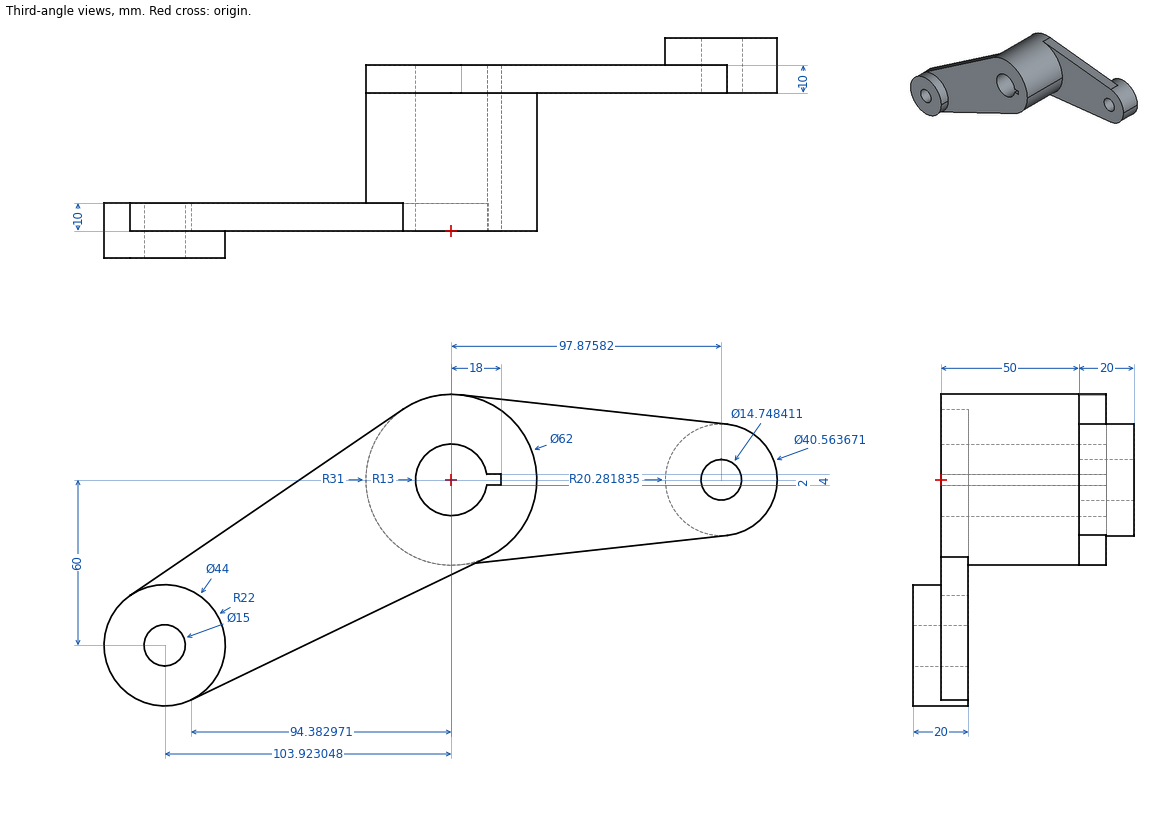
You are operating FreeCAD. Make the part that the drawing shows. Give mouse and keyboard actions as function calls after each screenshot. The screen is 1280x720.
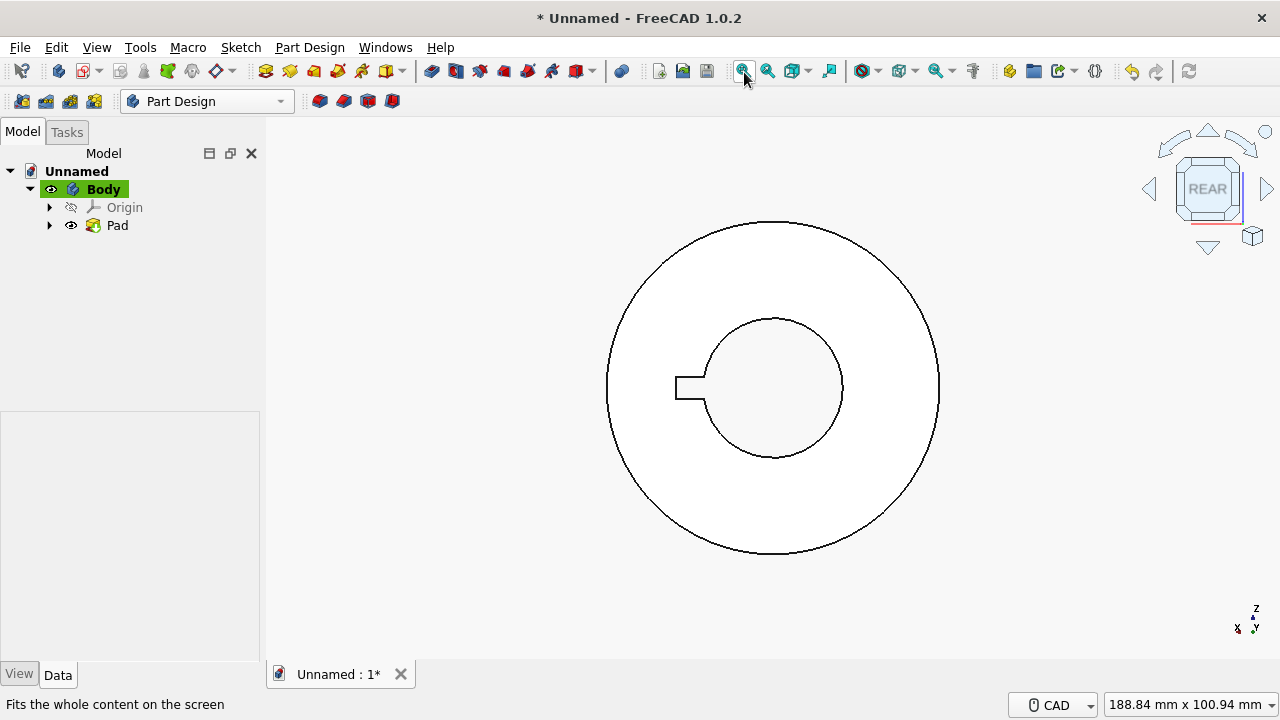
click(821, 292)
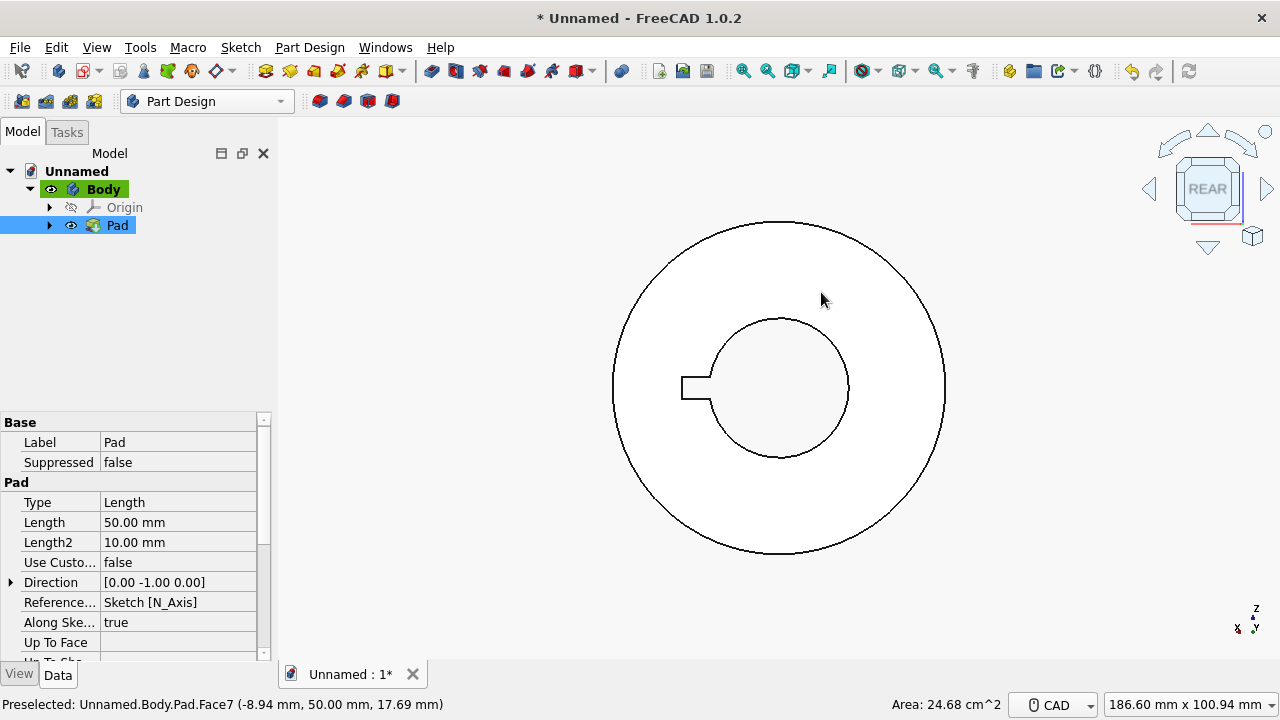
click(84, 72)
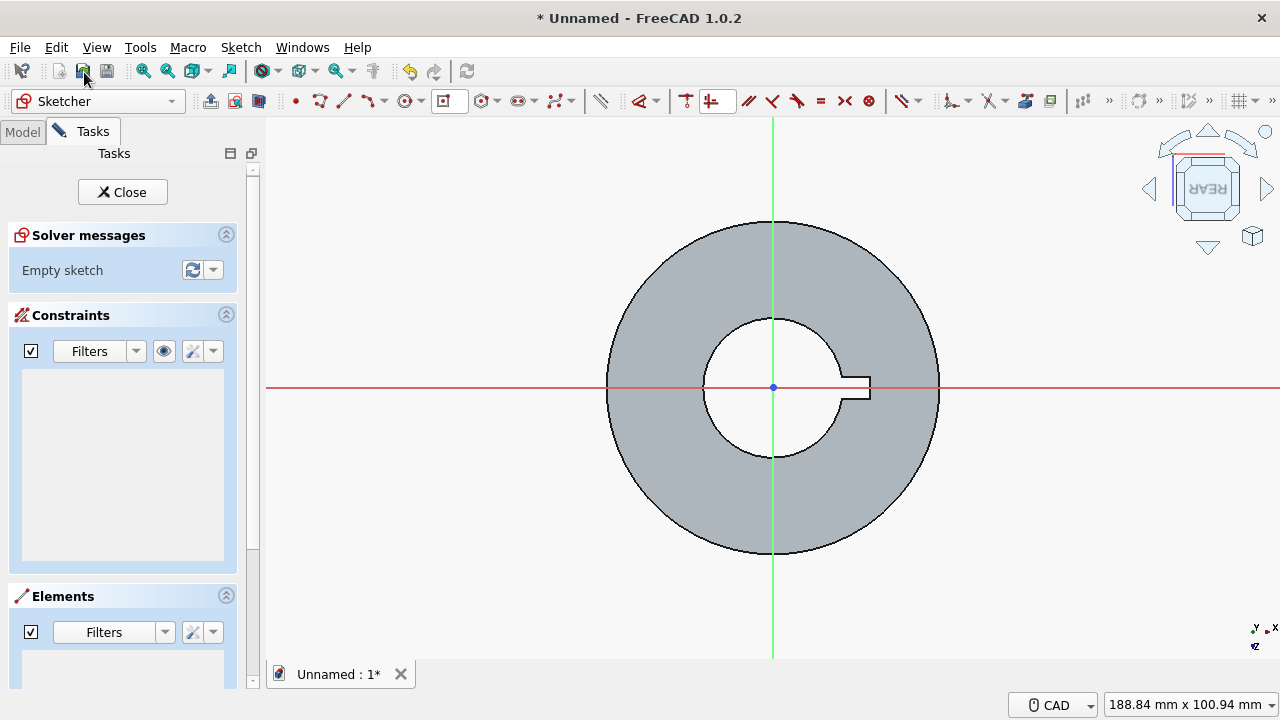
scroll(294, 388, down, 2)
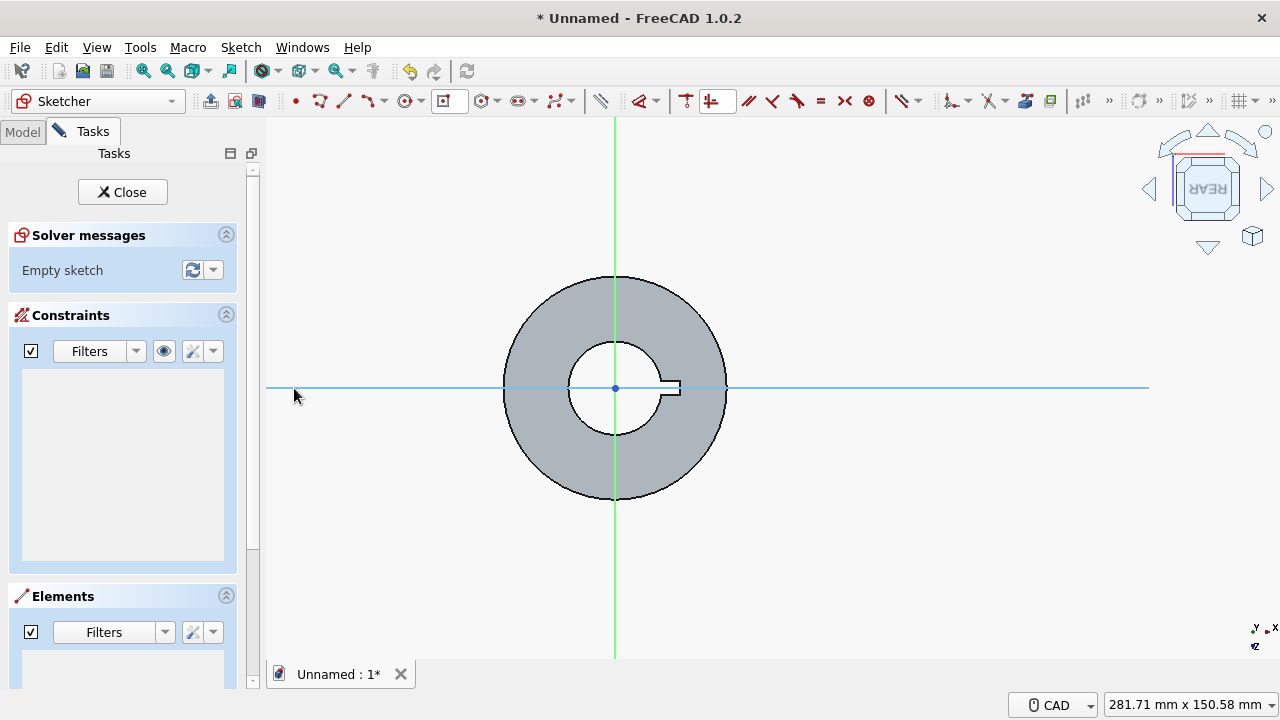
click(344, 102)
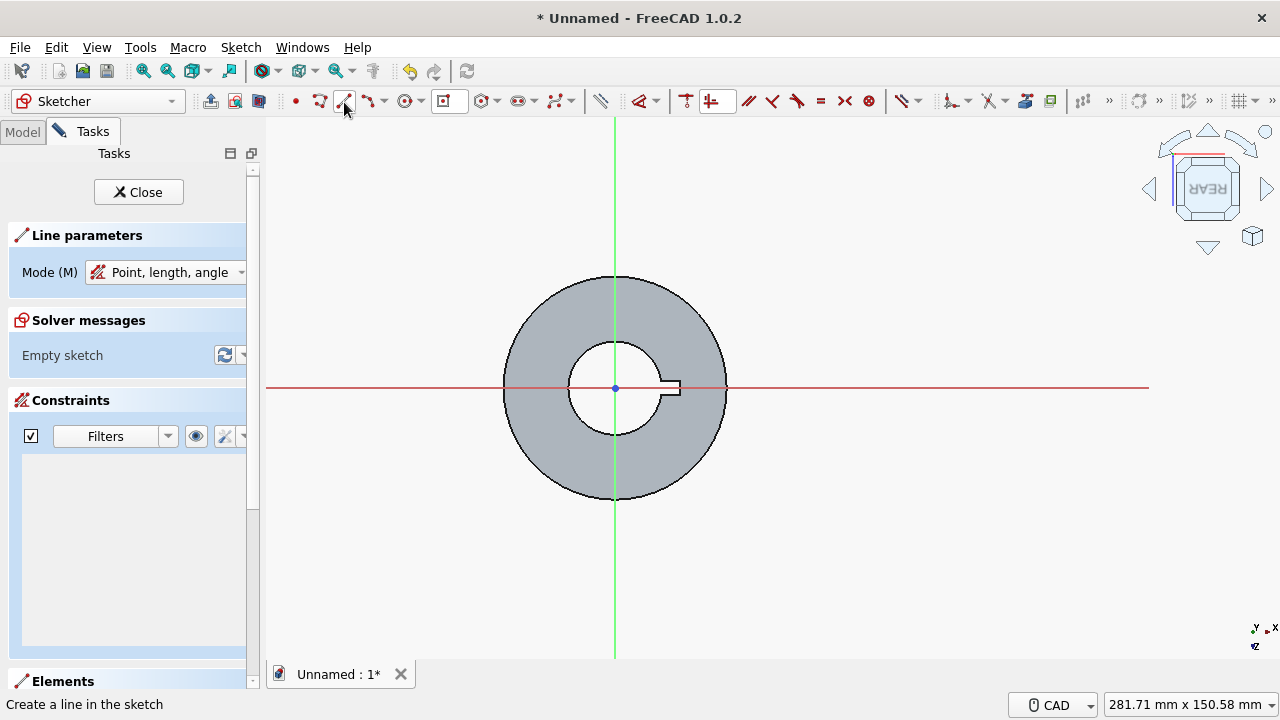
scroll(627, 499, up, 2)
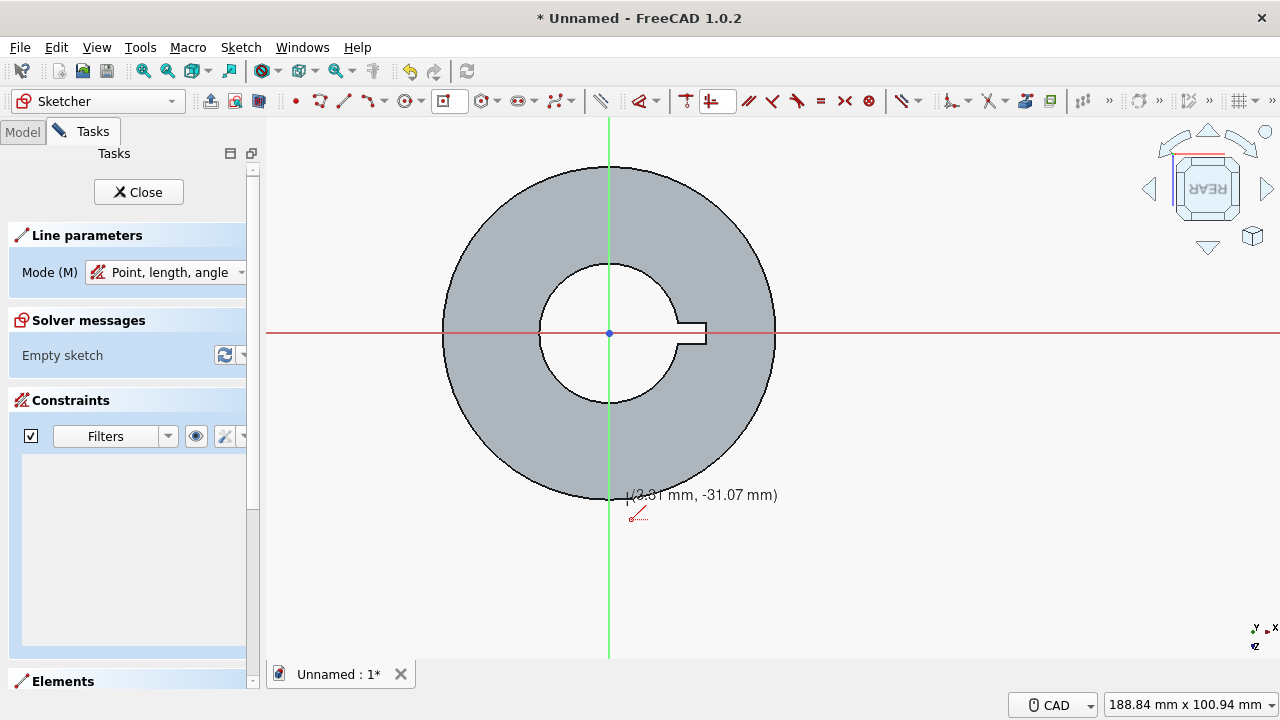
click(627, 499)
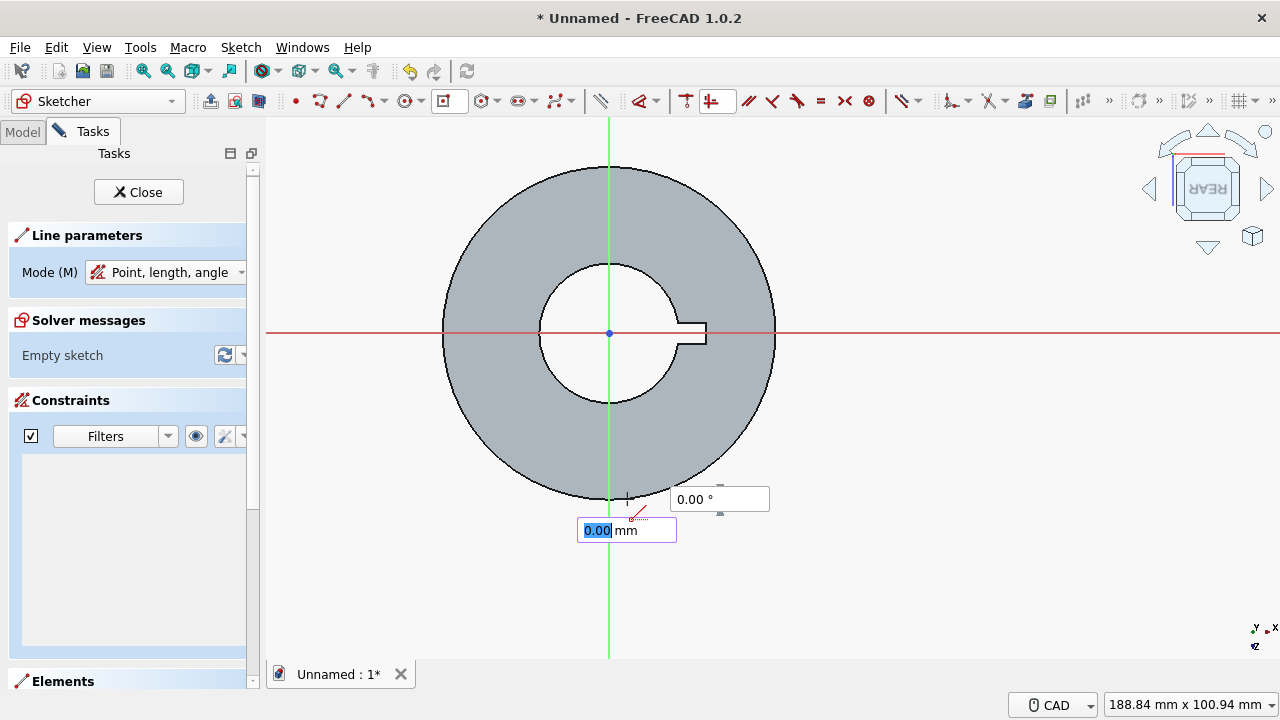
scroll(298, 631, down, 1)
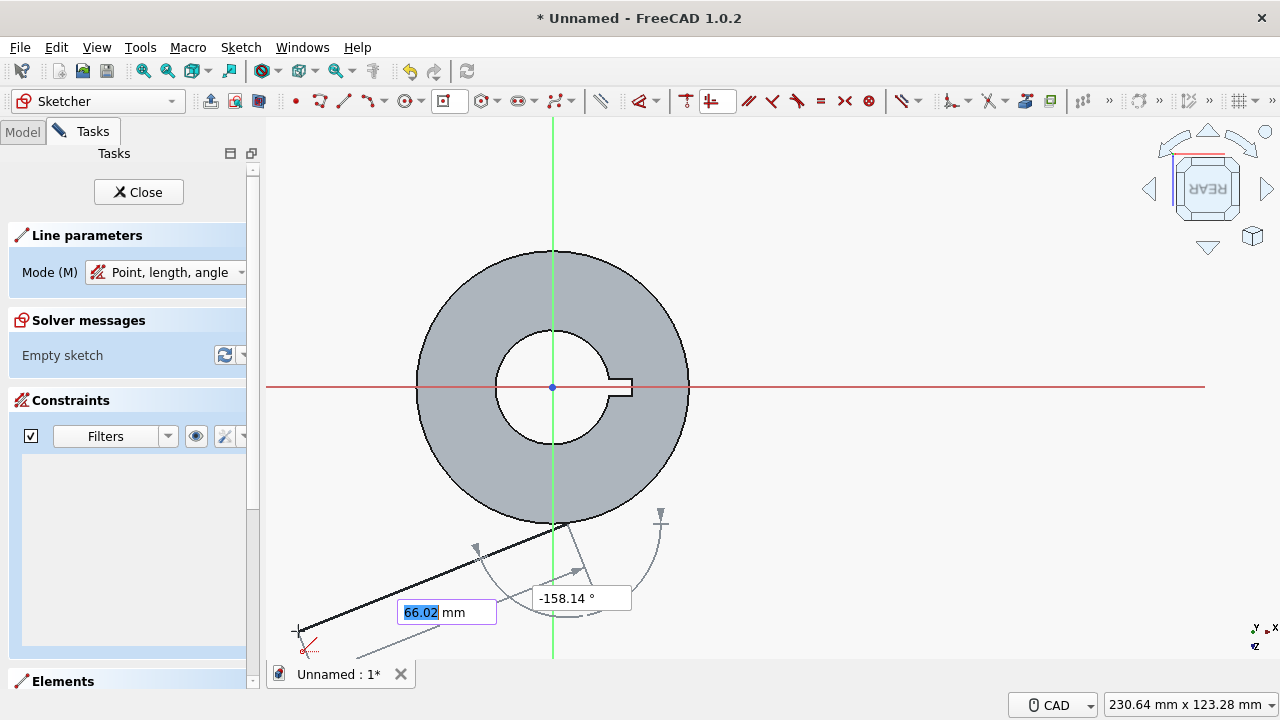
click(993, 476)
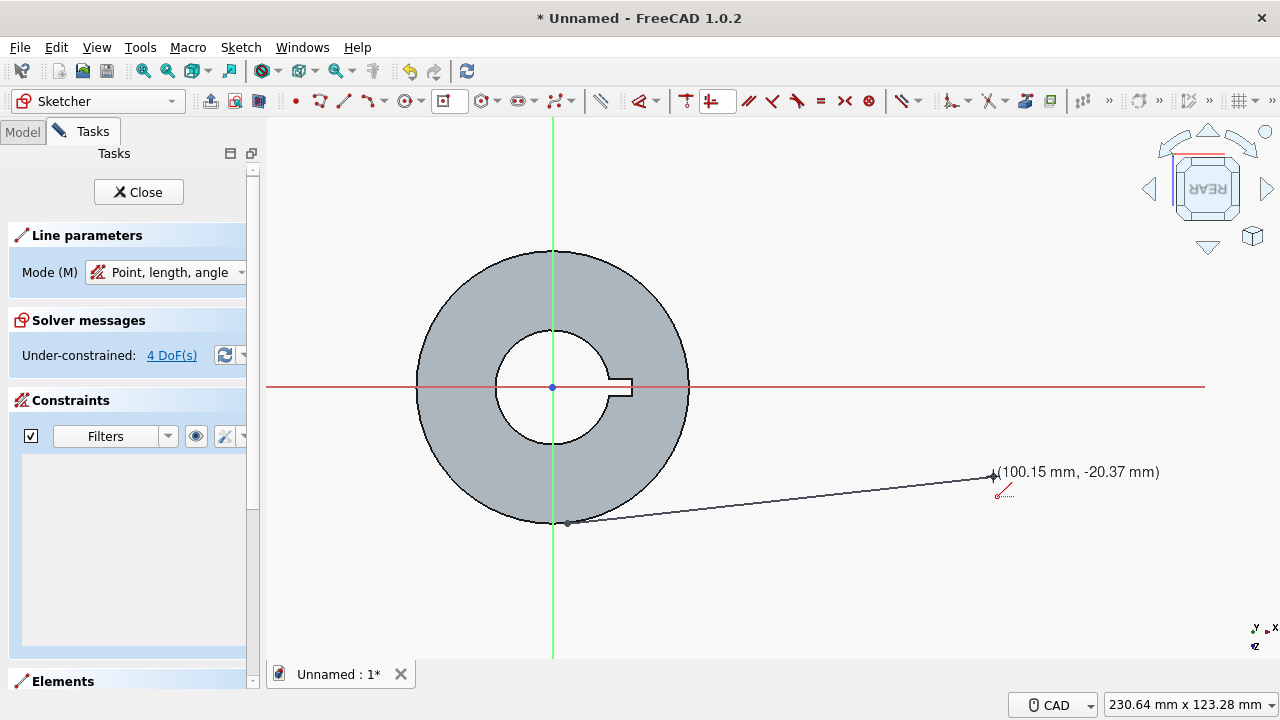
click(993, 299)
click(568, 252)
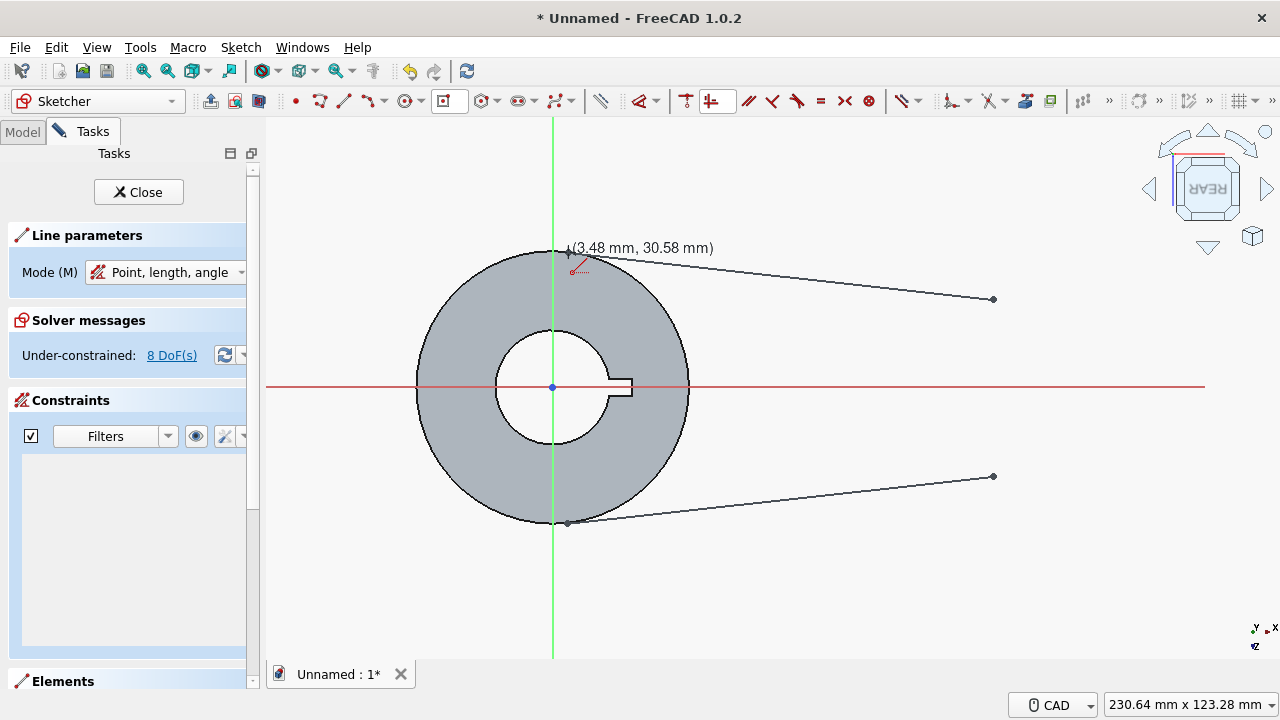
click(368, 102)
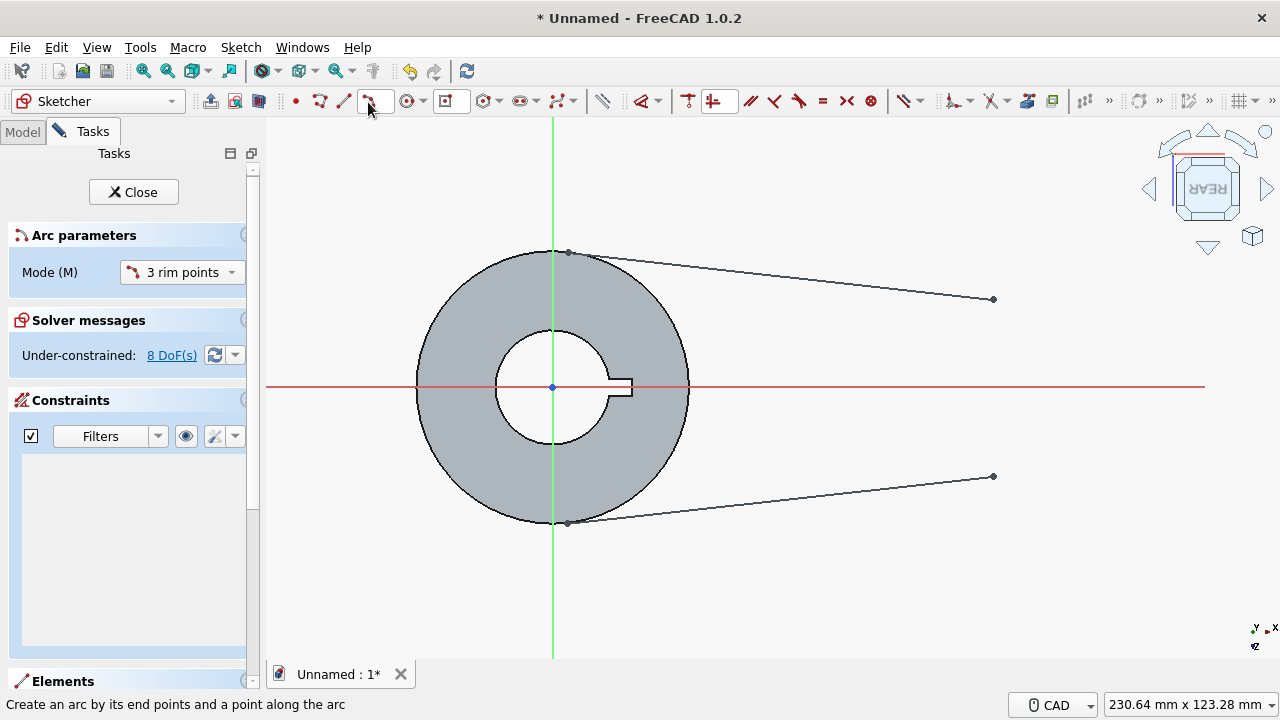
click(993, 477)
click(993, 300)
click(899, 358)